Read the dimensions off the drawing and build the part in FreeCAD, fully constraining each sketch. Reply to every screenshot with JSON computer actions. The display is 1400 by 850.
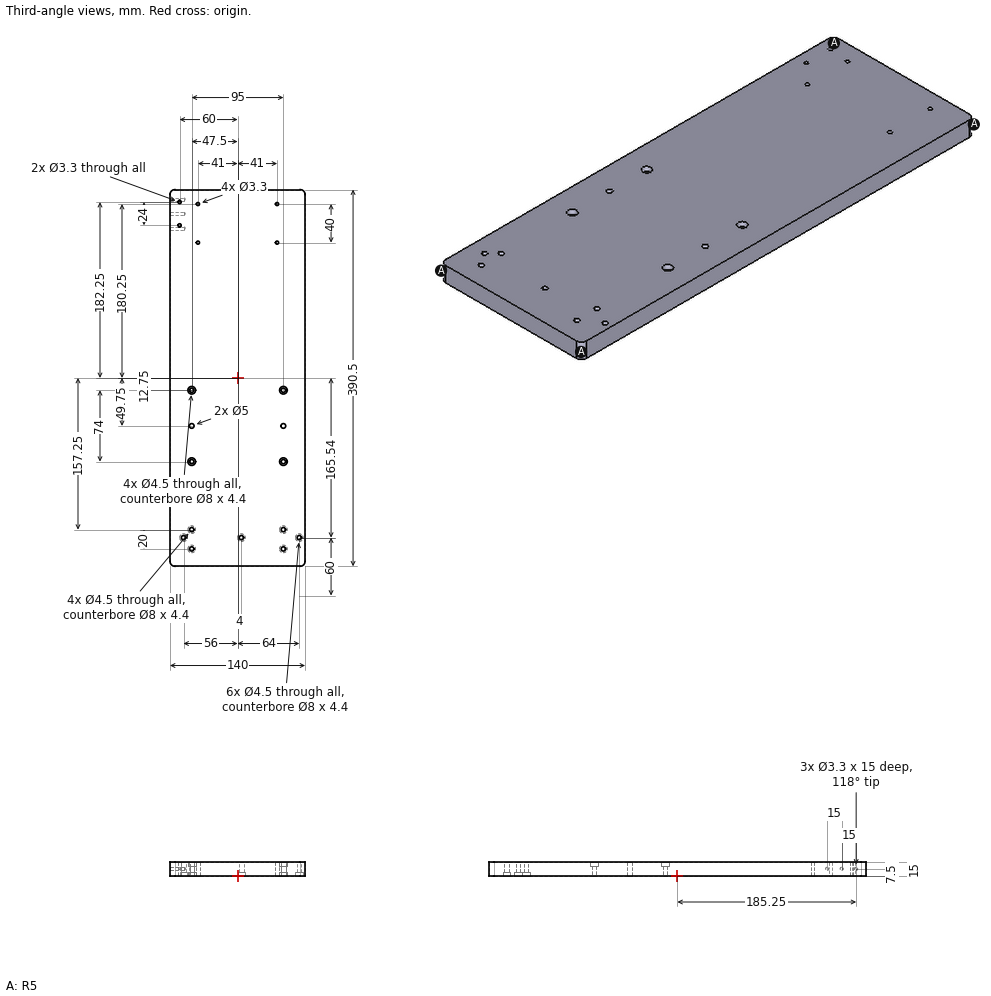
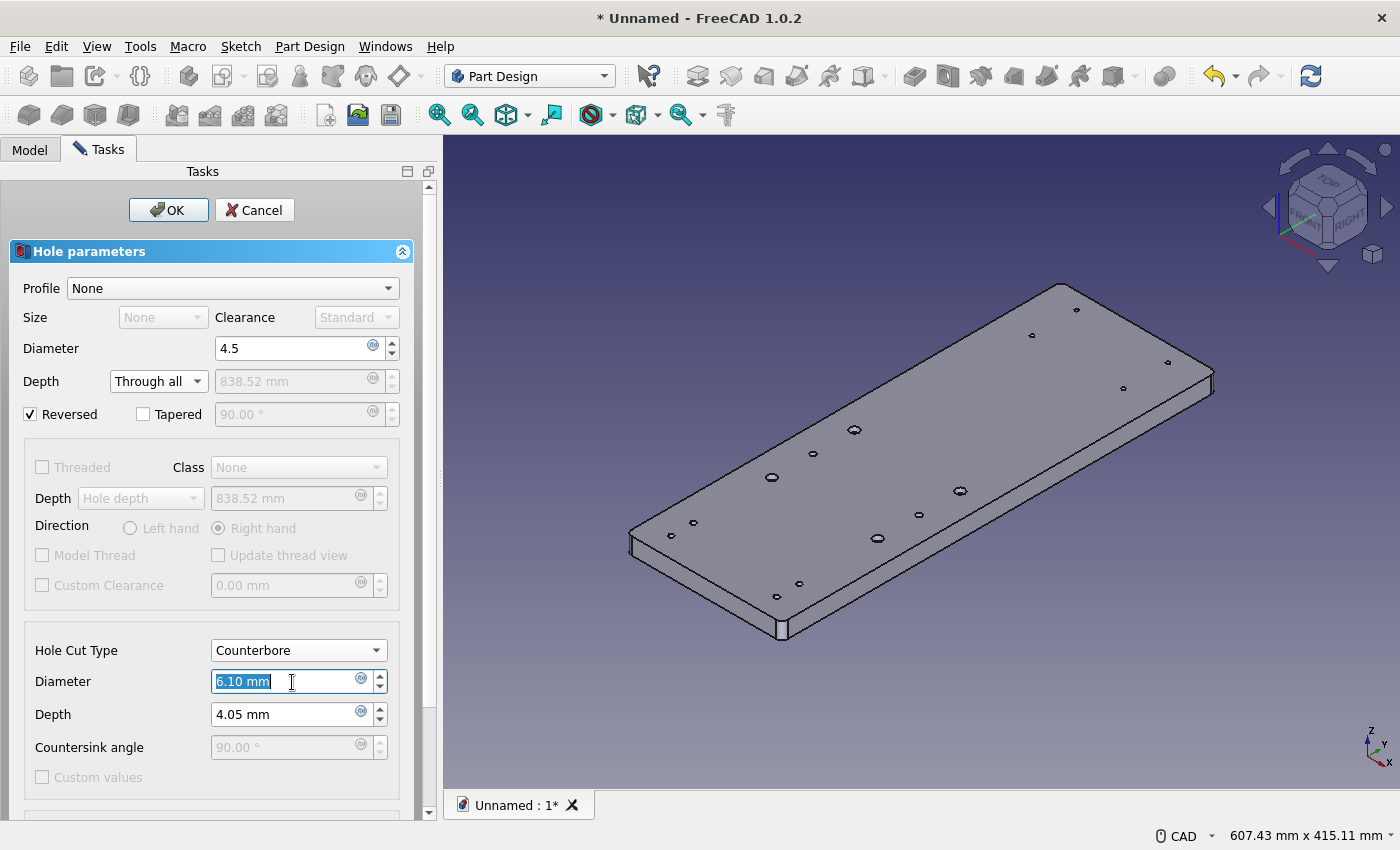
{"action": "type", "text": "8"}
{"action": "key", "text": "Tab"}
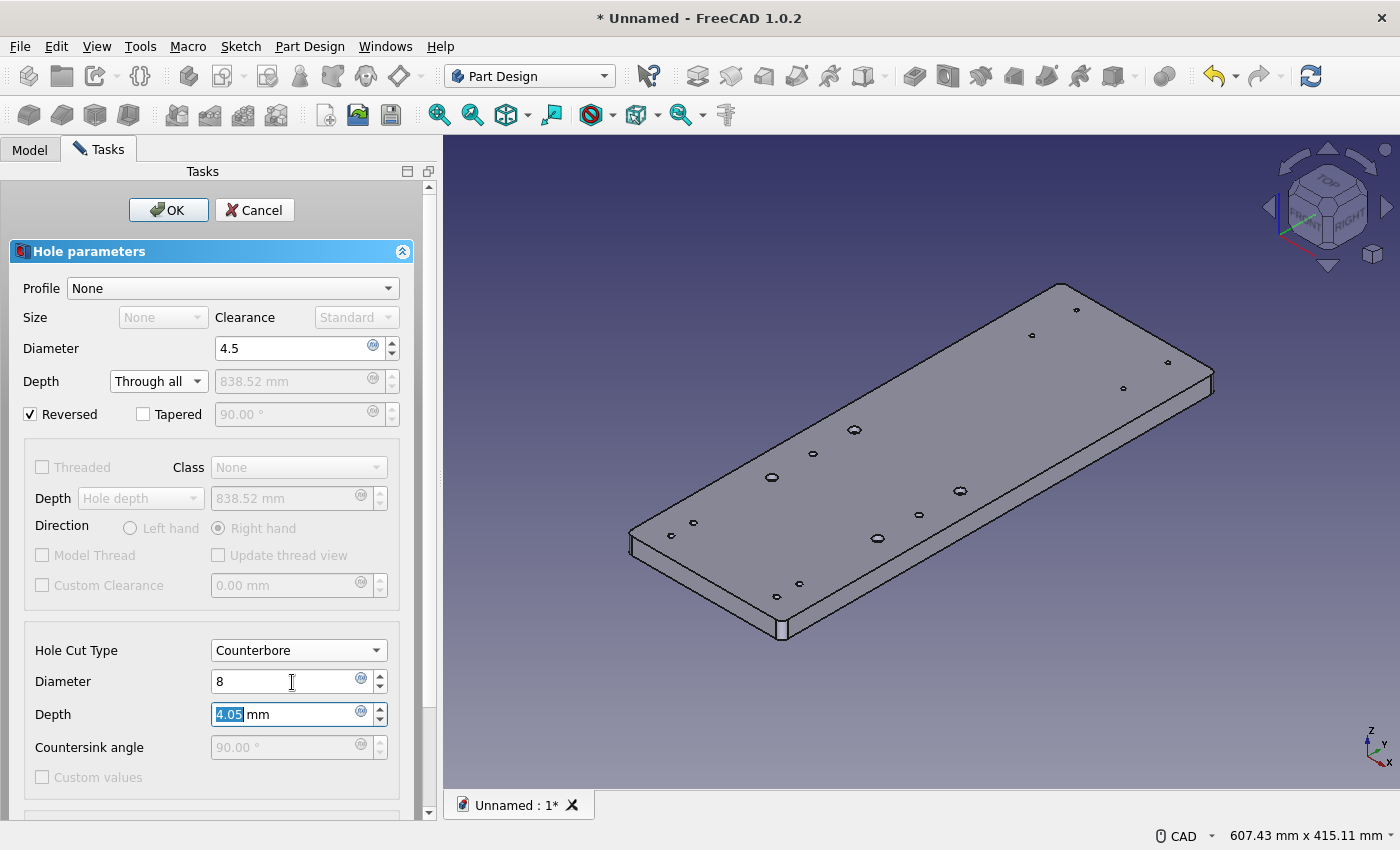
{"action": "type", "text": "4.4"}
{"action": "key", "text": "Tab"}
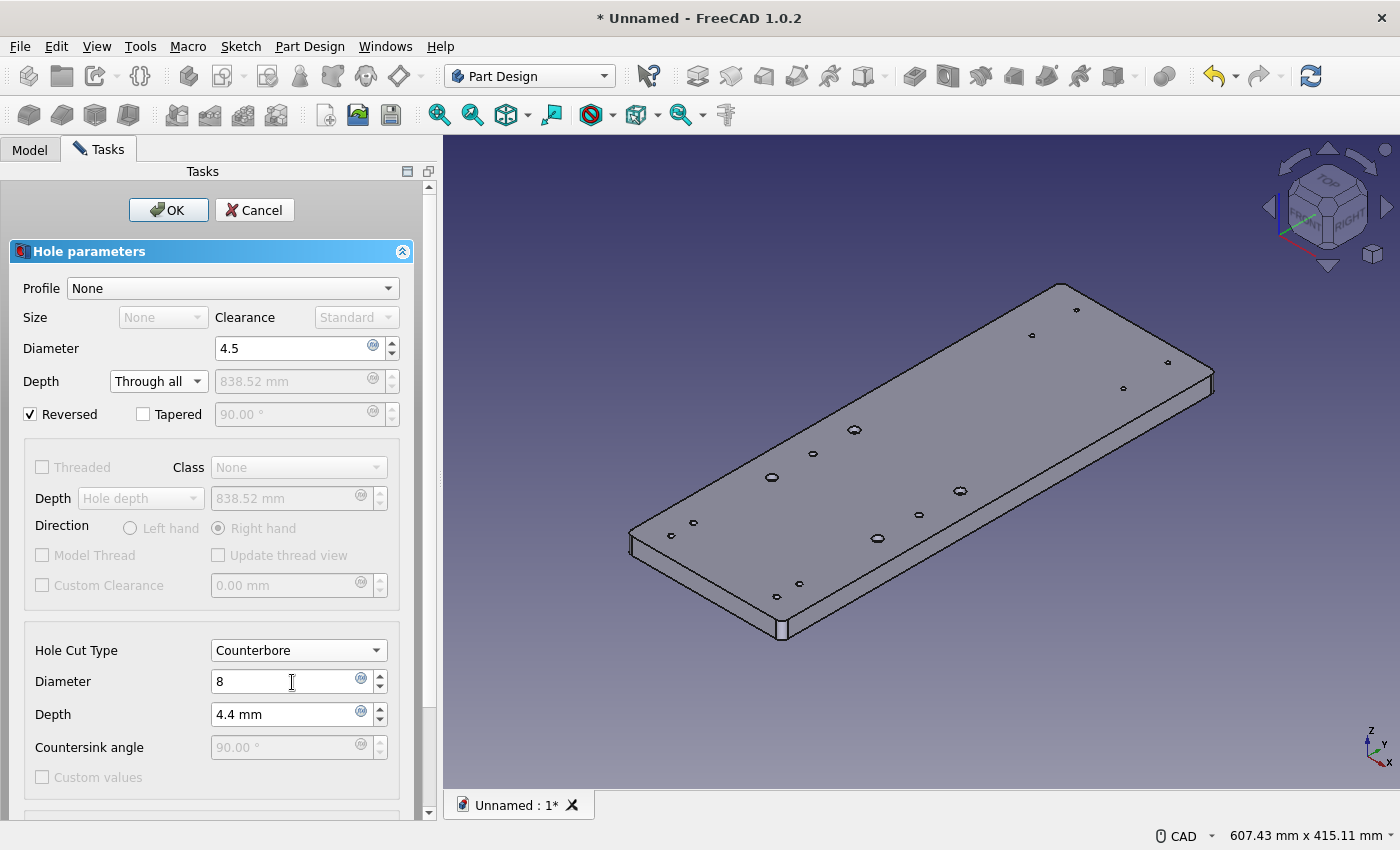
{"action": "left_click", "coordinate": [169, 210]}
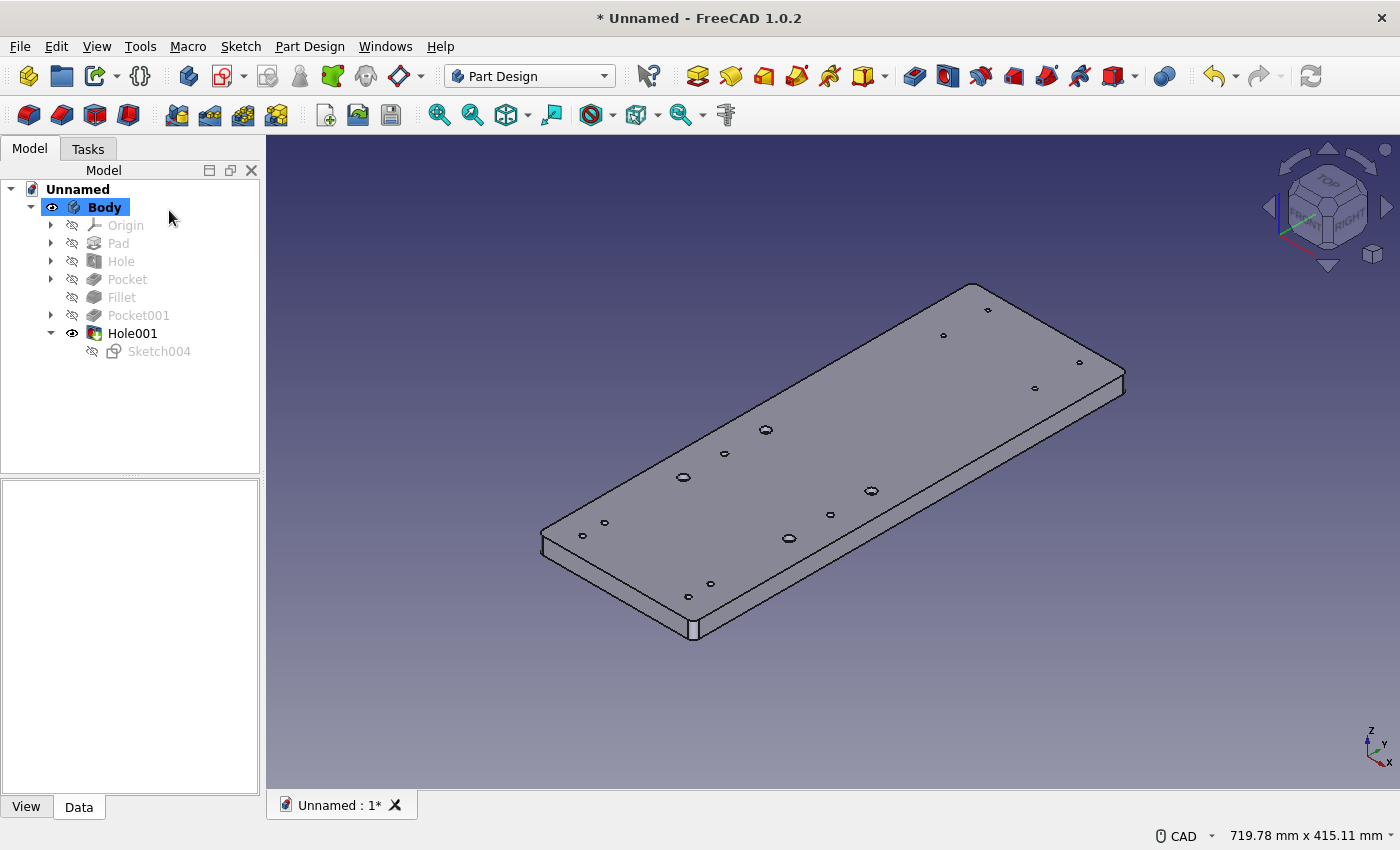
{"action": "key", "text": "6"}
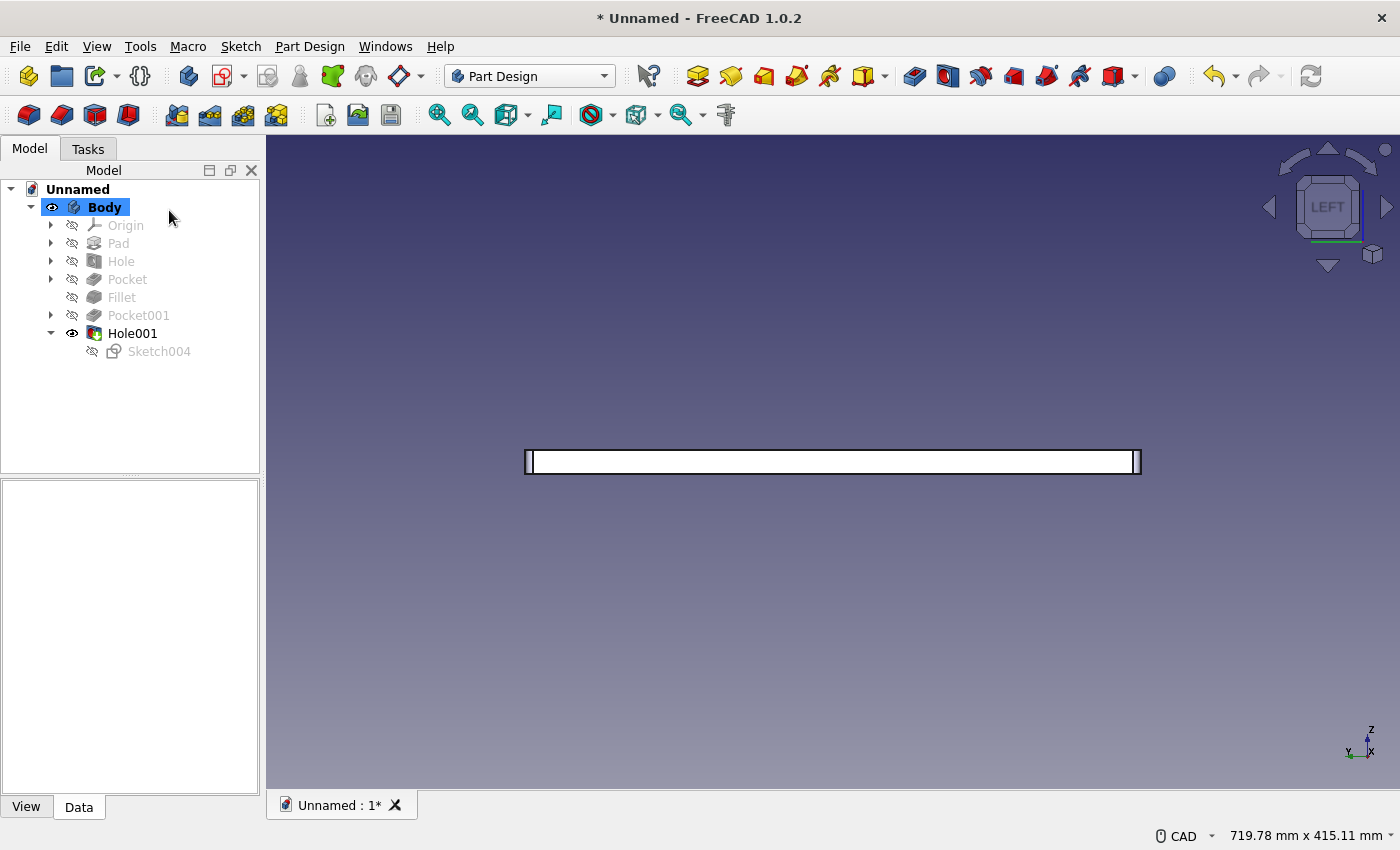
{"action": "left_click", "coordinate": [576, 461]}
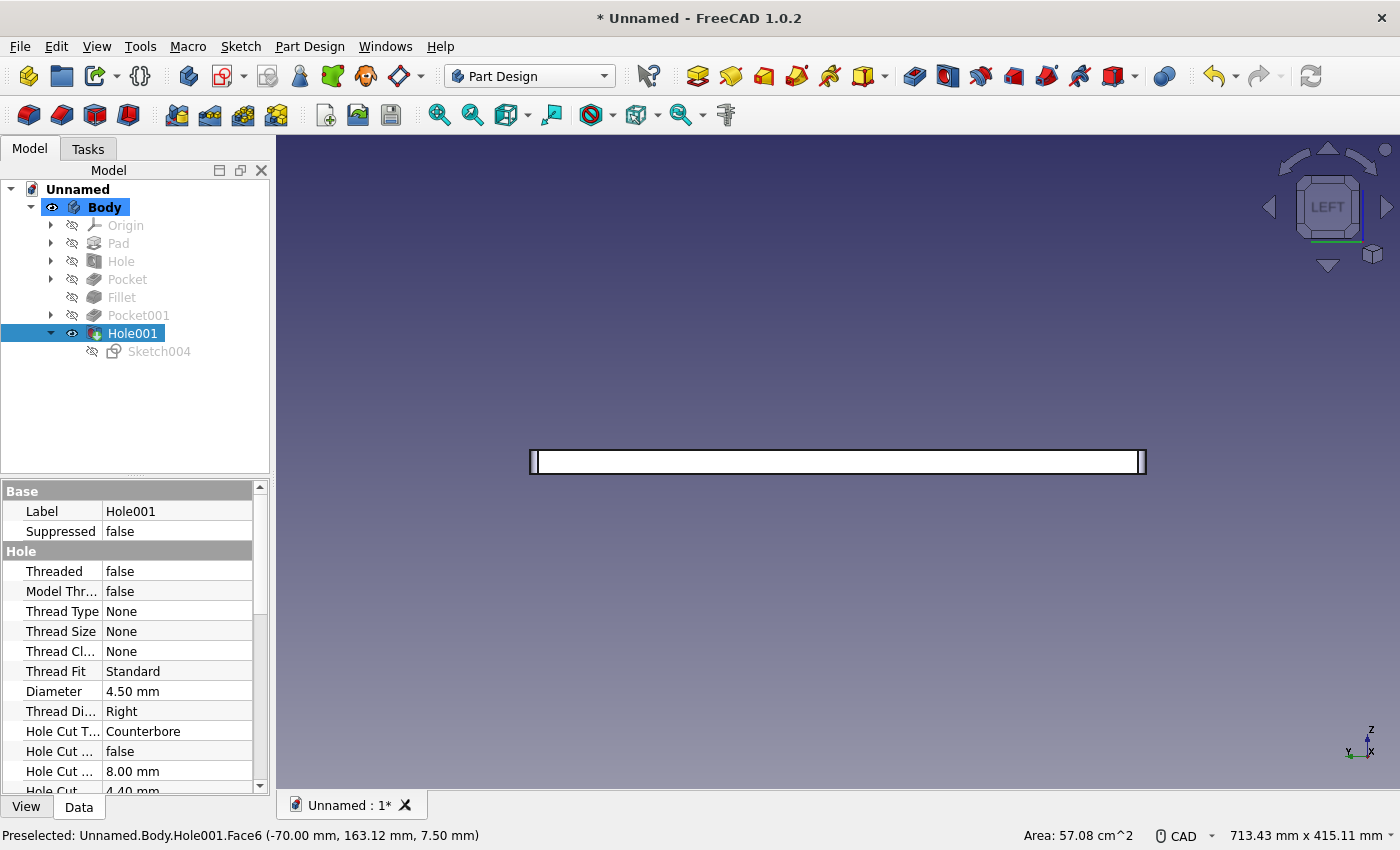
{"action": "left_click", "coordinate": [222, 76]}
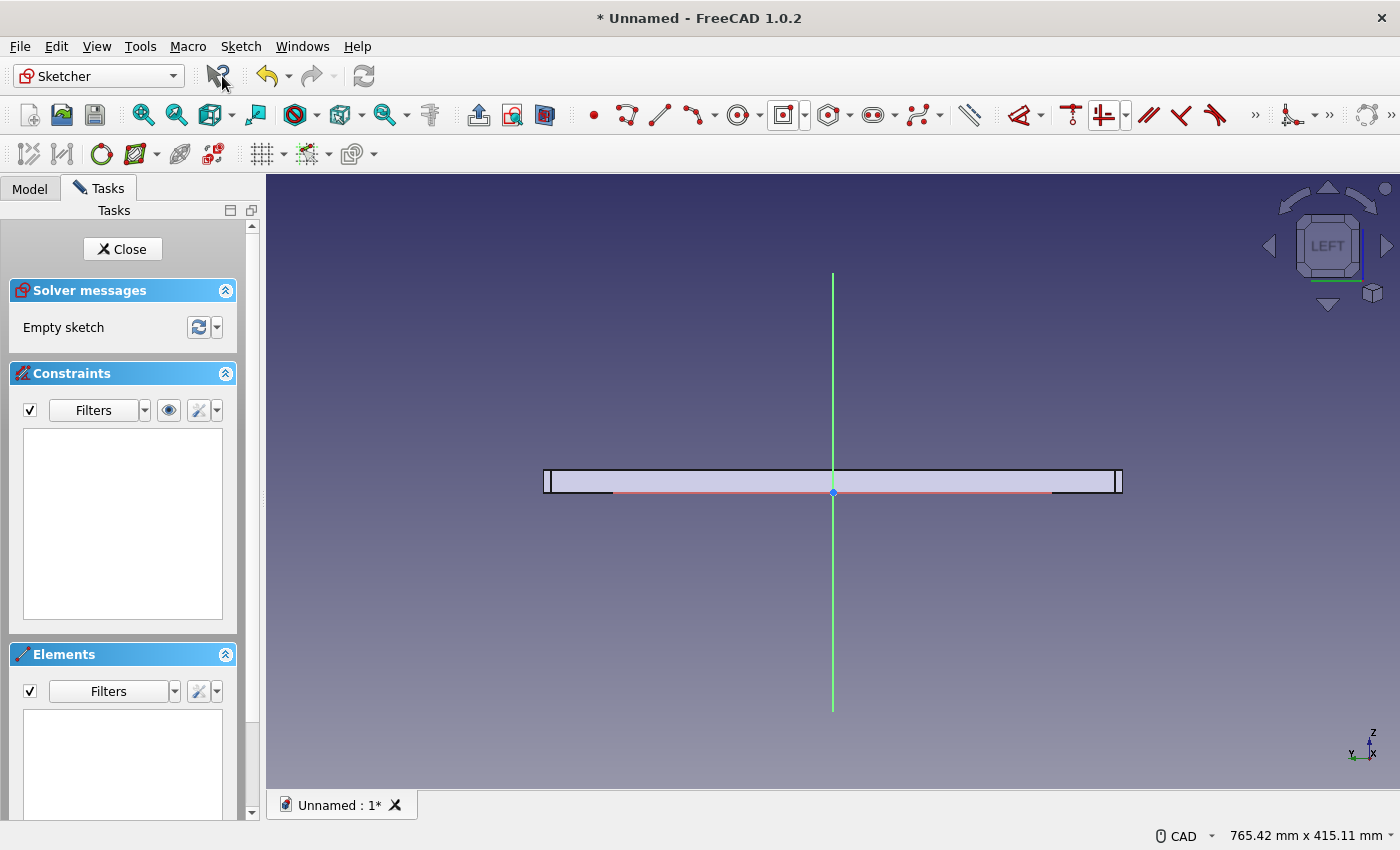
{"action": "scroll", "coordinate": [566, 482], "scroll_direction": "up", "scroll_amount": 13}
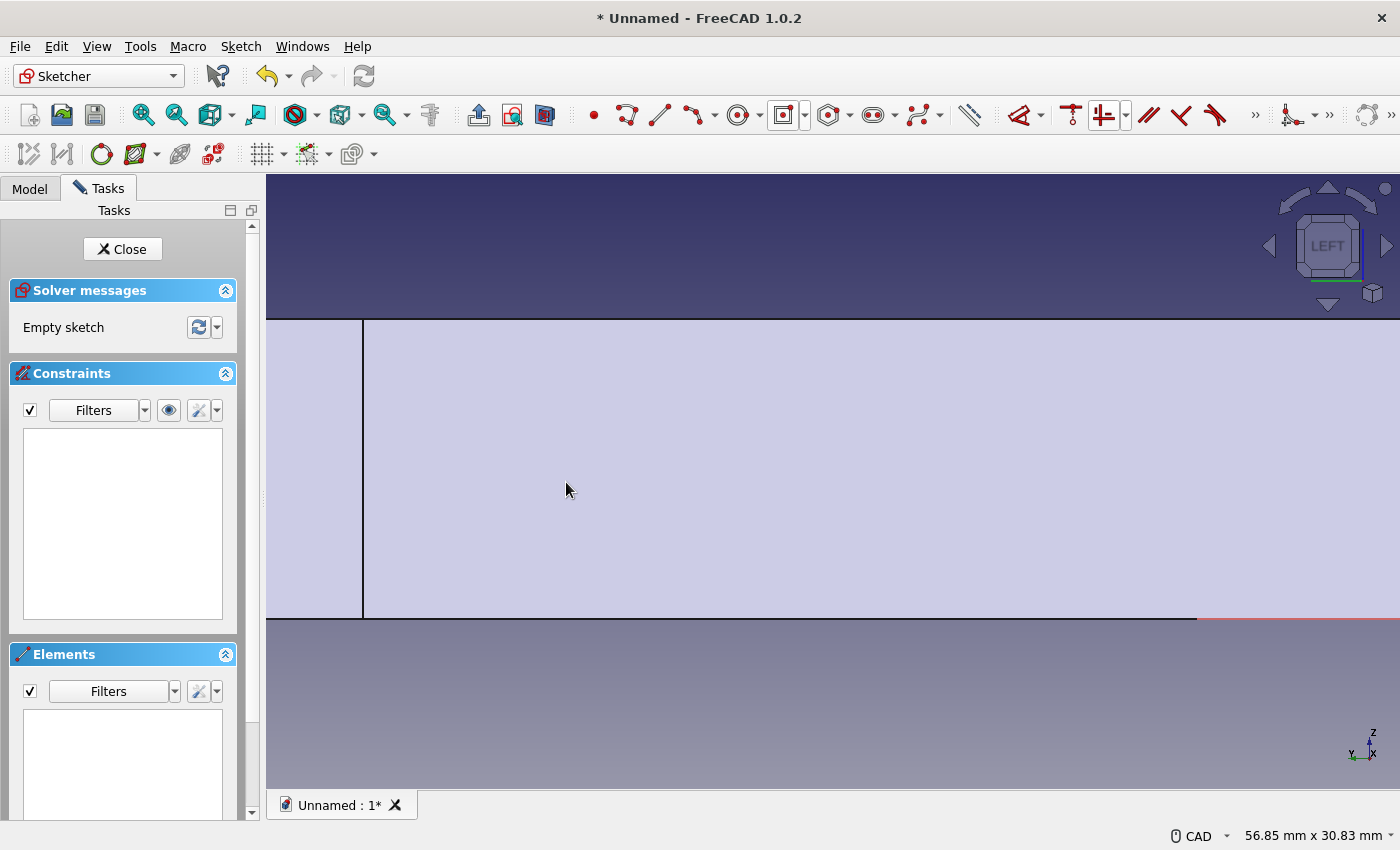
{"action": "left_click", "coordinate": [738, 116]}